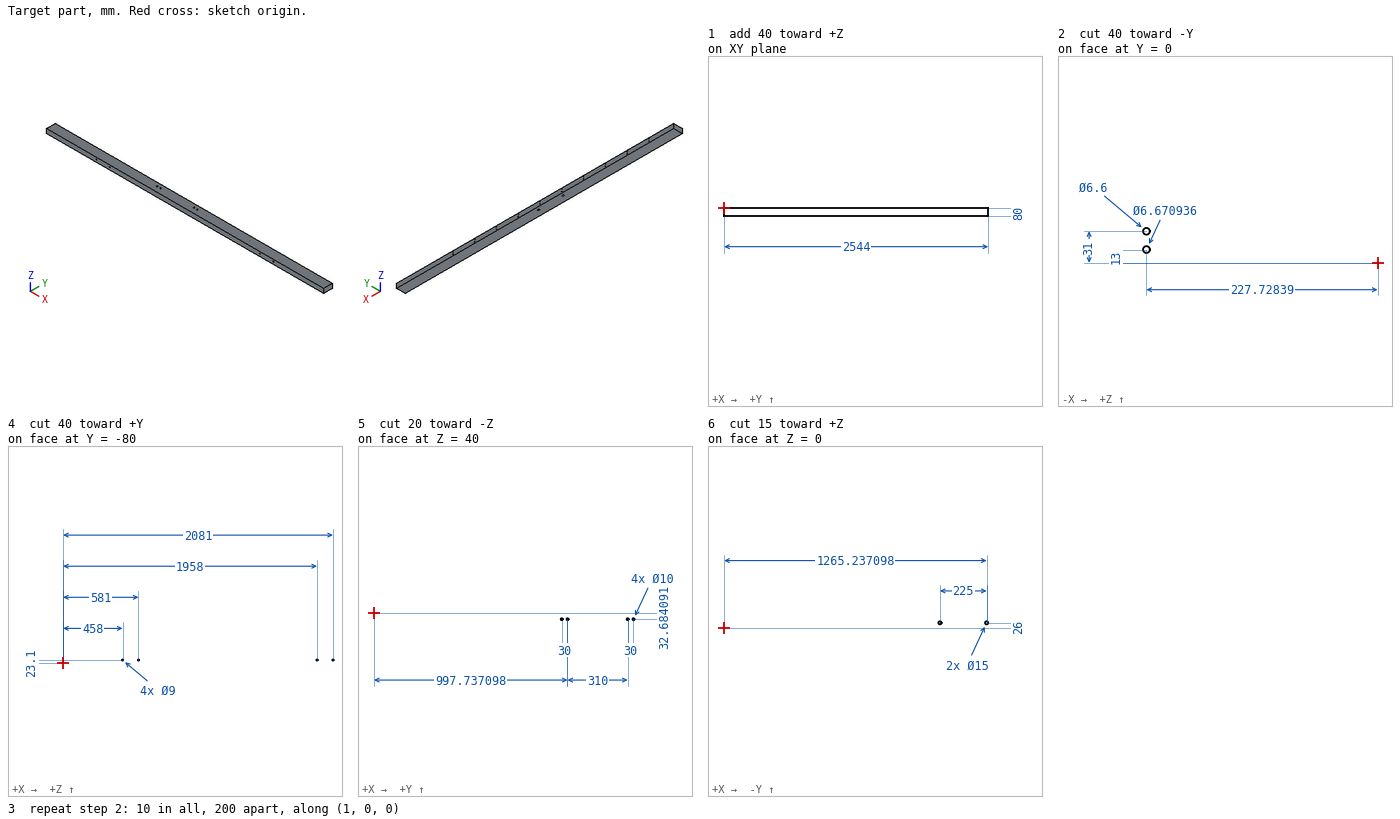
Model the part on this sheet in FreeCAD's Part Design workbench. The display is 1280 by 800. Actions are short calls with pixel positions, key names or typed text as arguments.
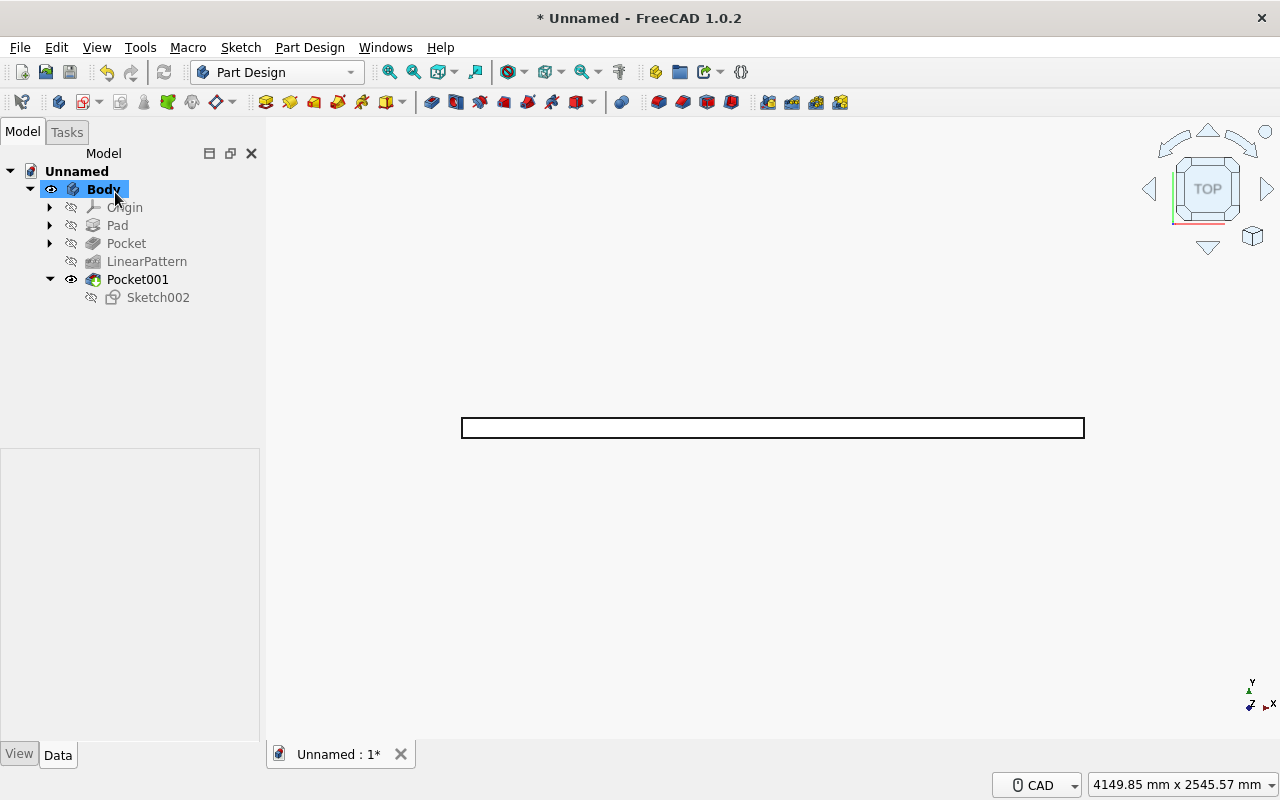
click(1039, 427)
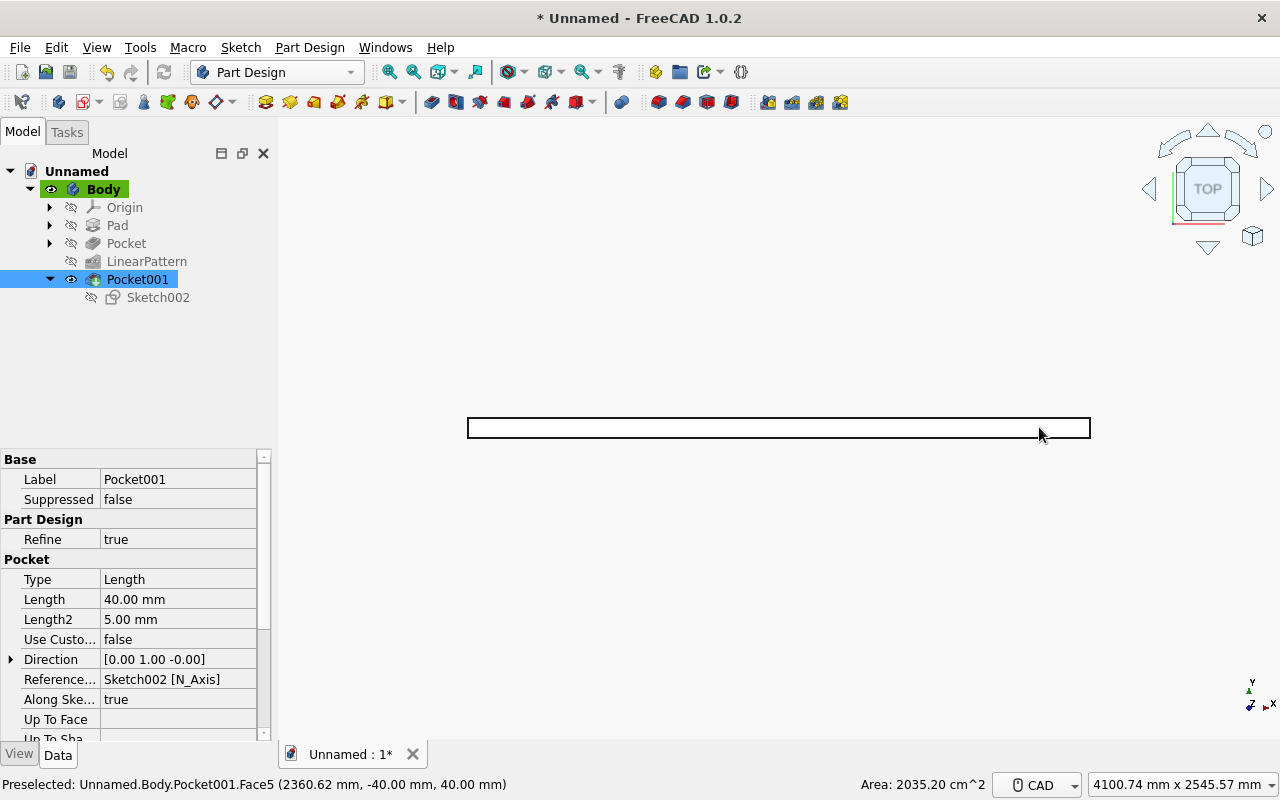
click(84, 102)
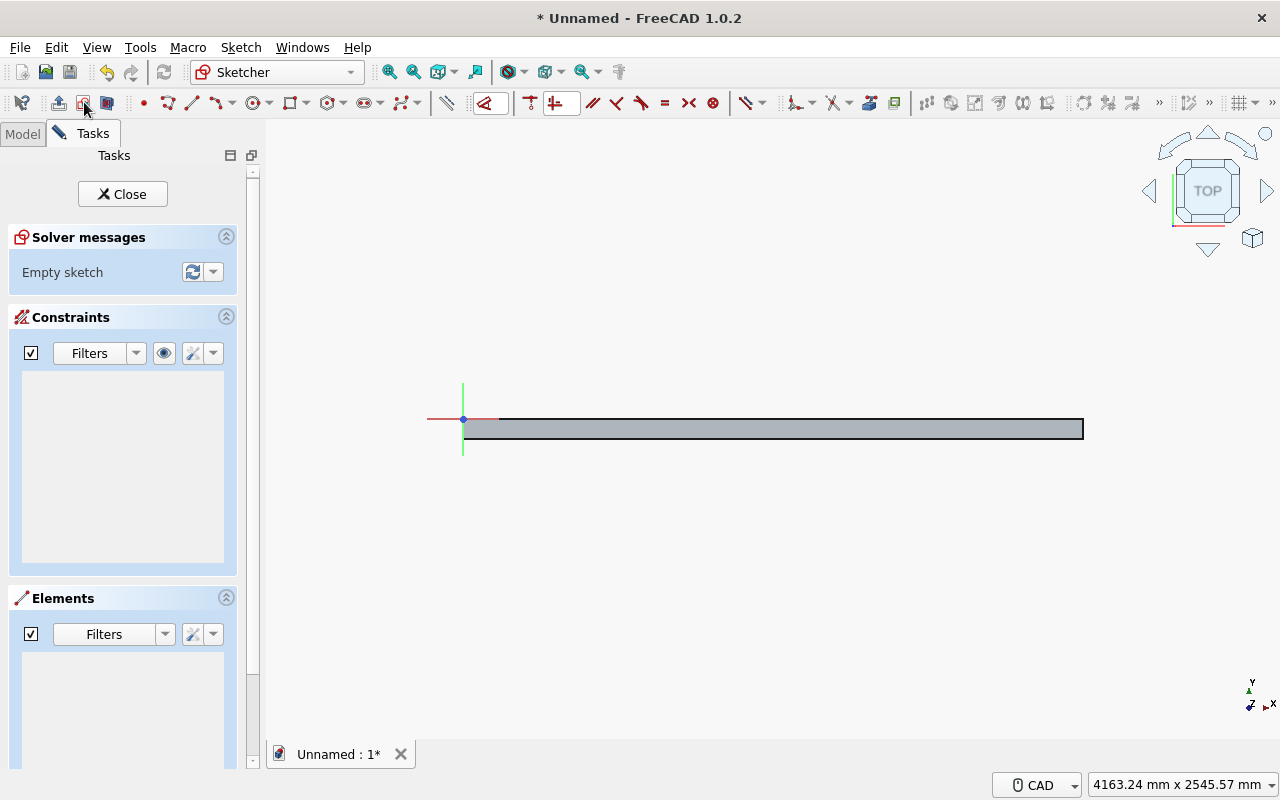
scroll(752, 427, up, 9)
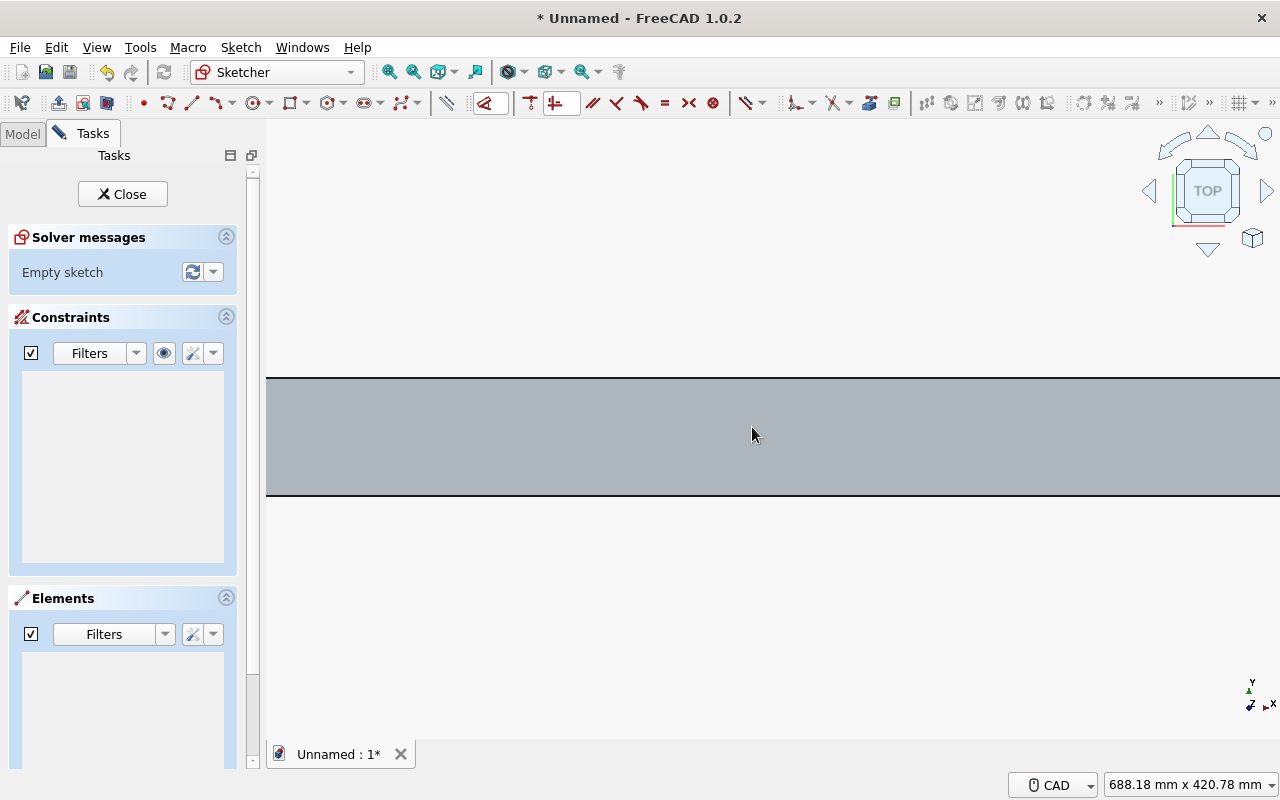
click(254, 104)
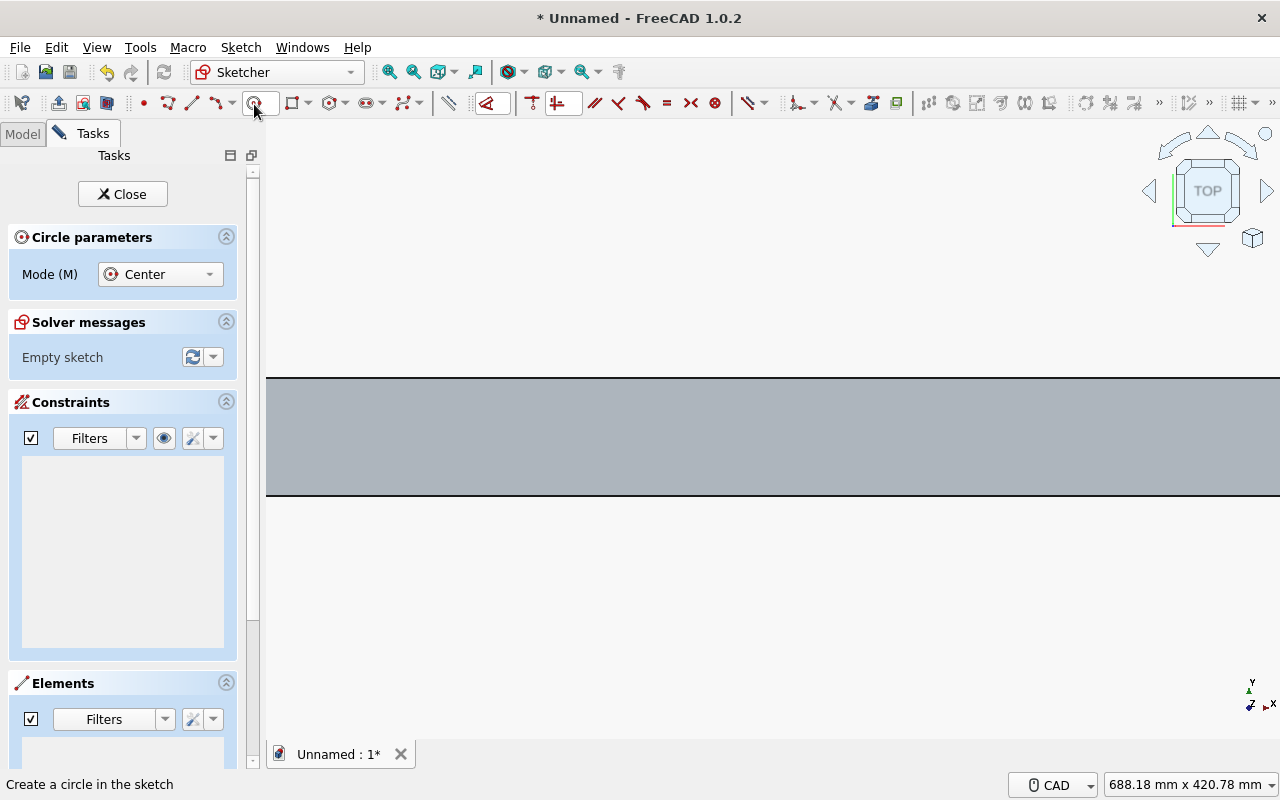
scroll(973, 426, up, 6)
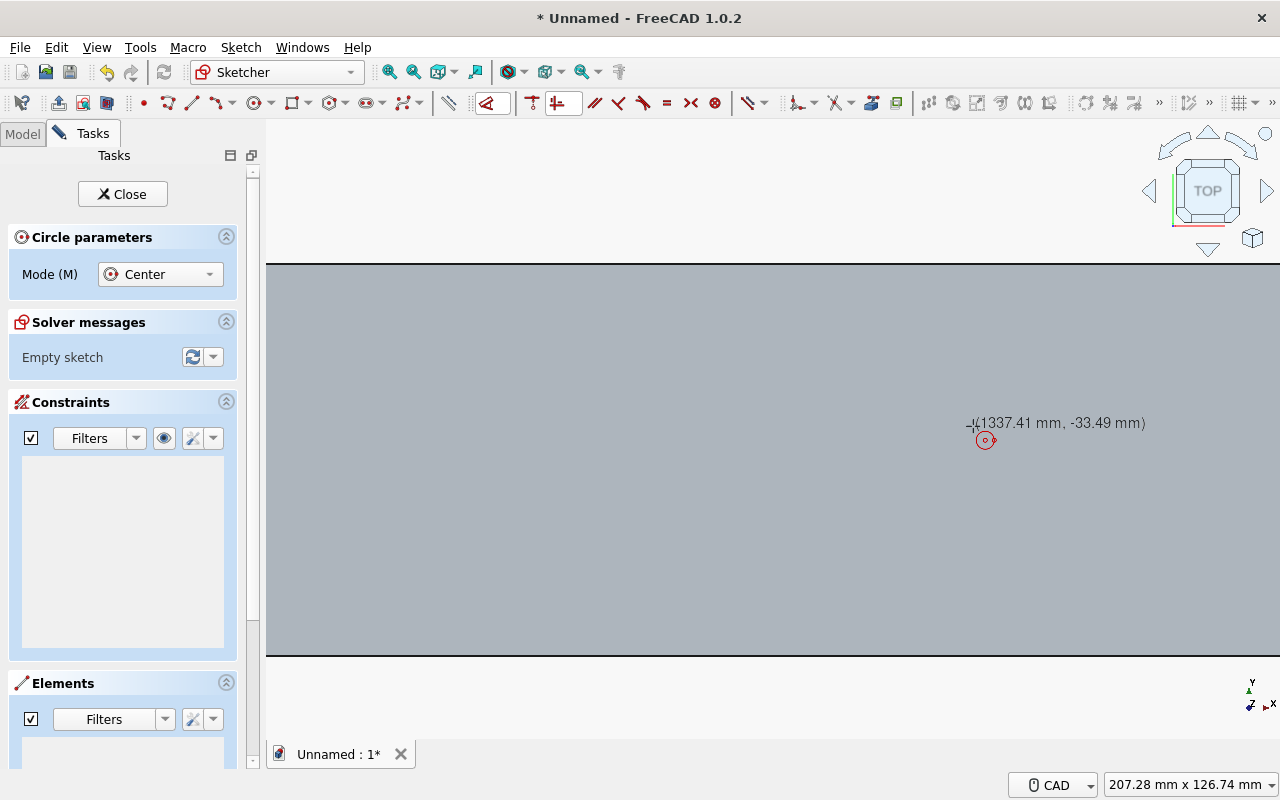
click(973, 424)
move(990, 407)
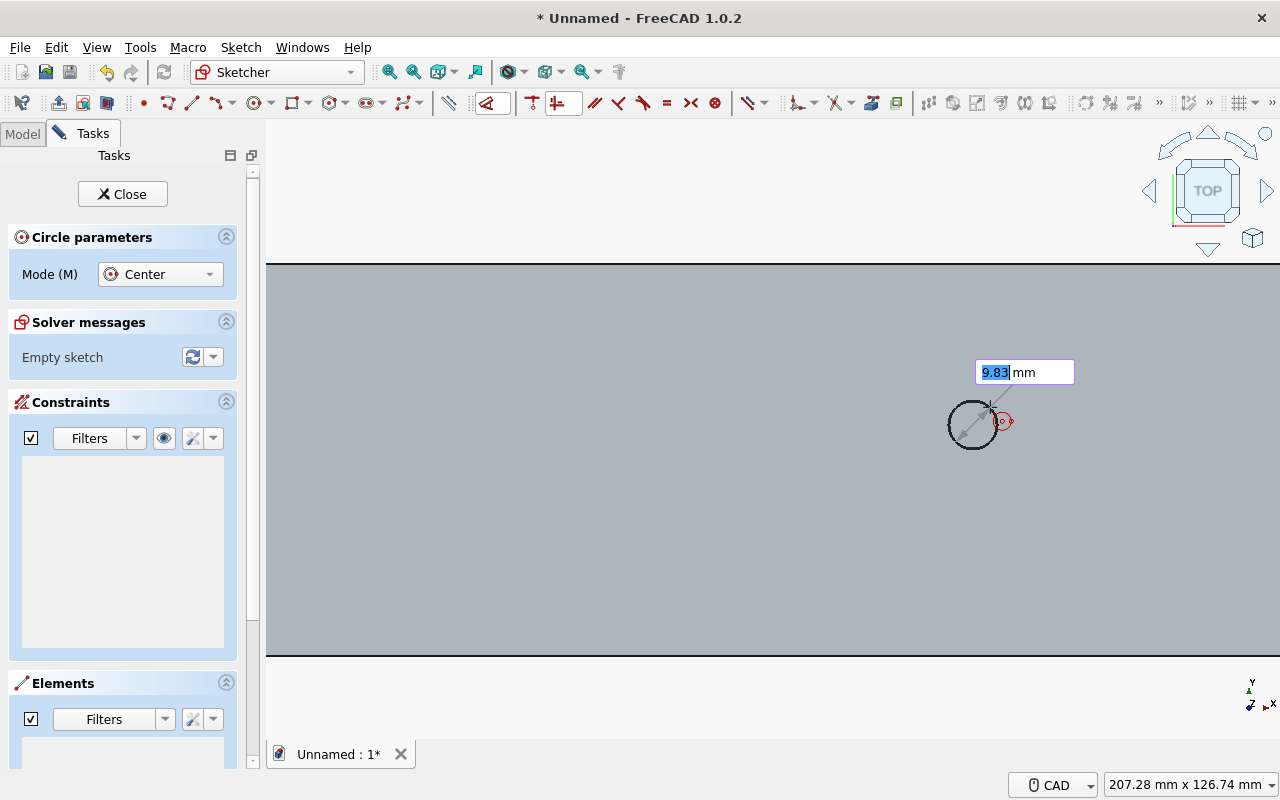
text(10)
key(Return)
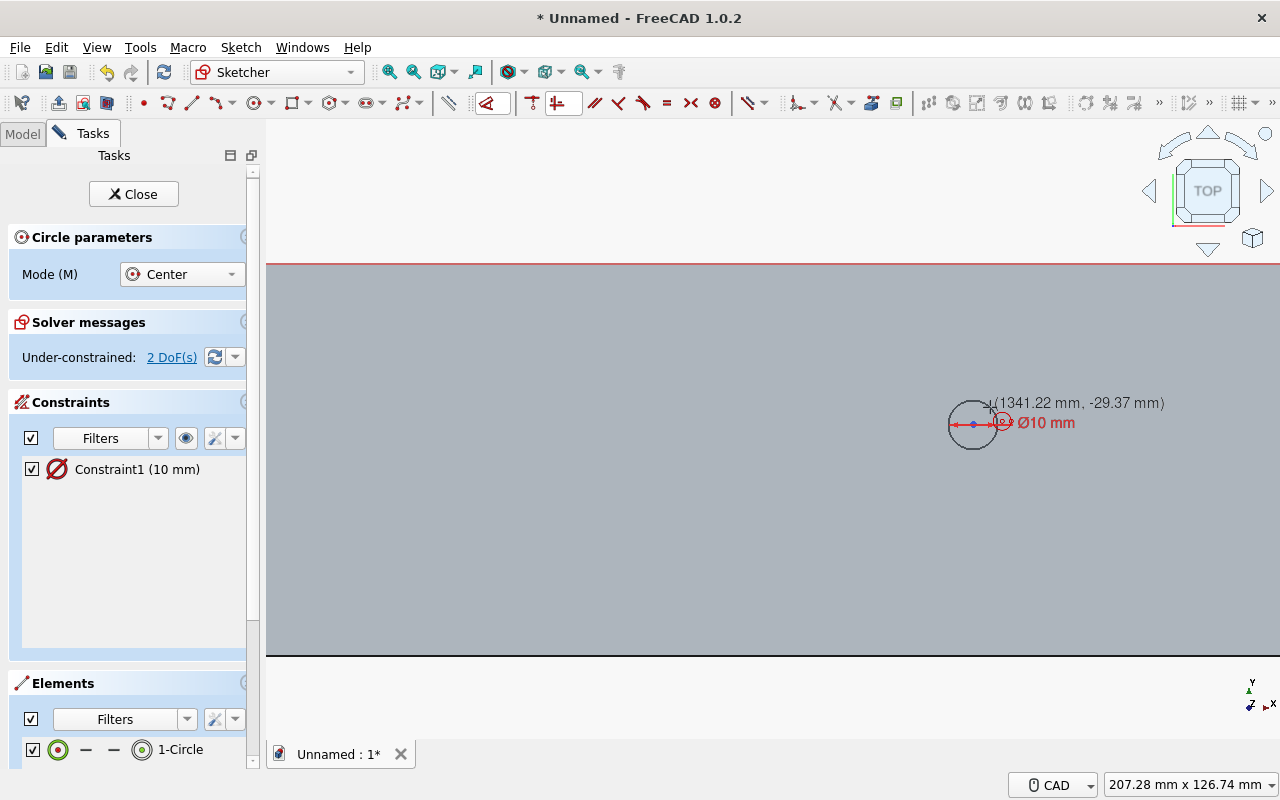
click(826, 424)
move(844, 407)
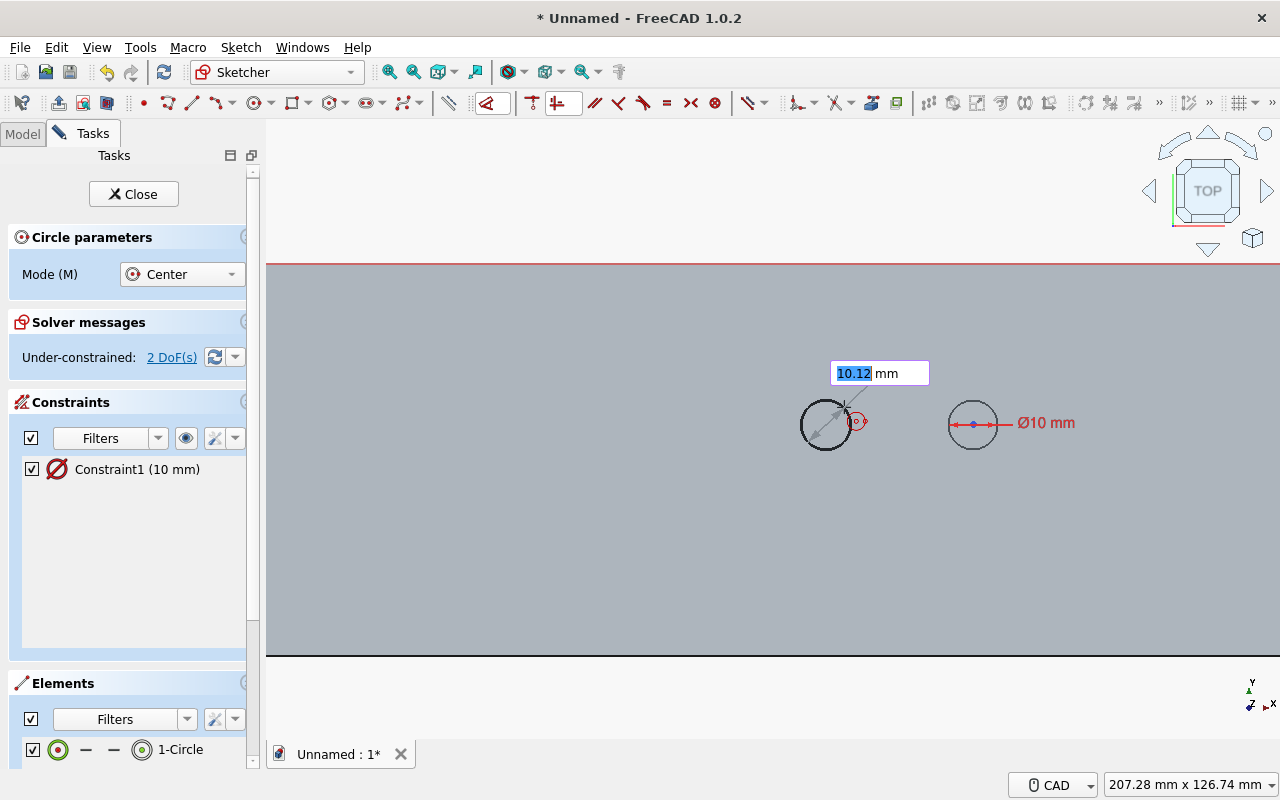
text(10)
key(Return)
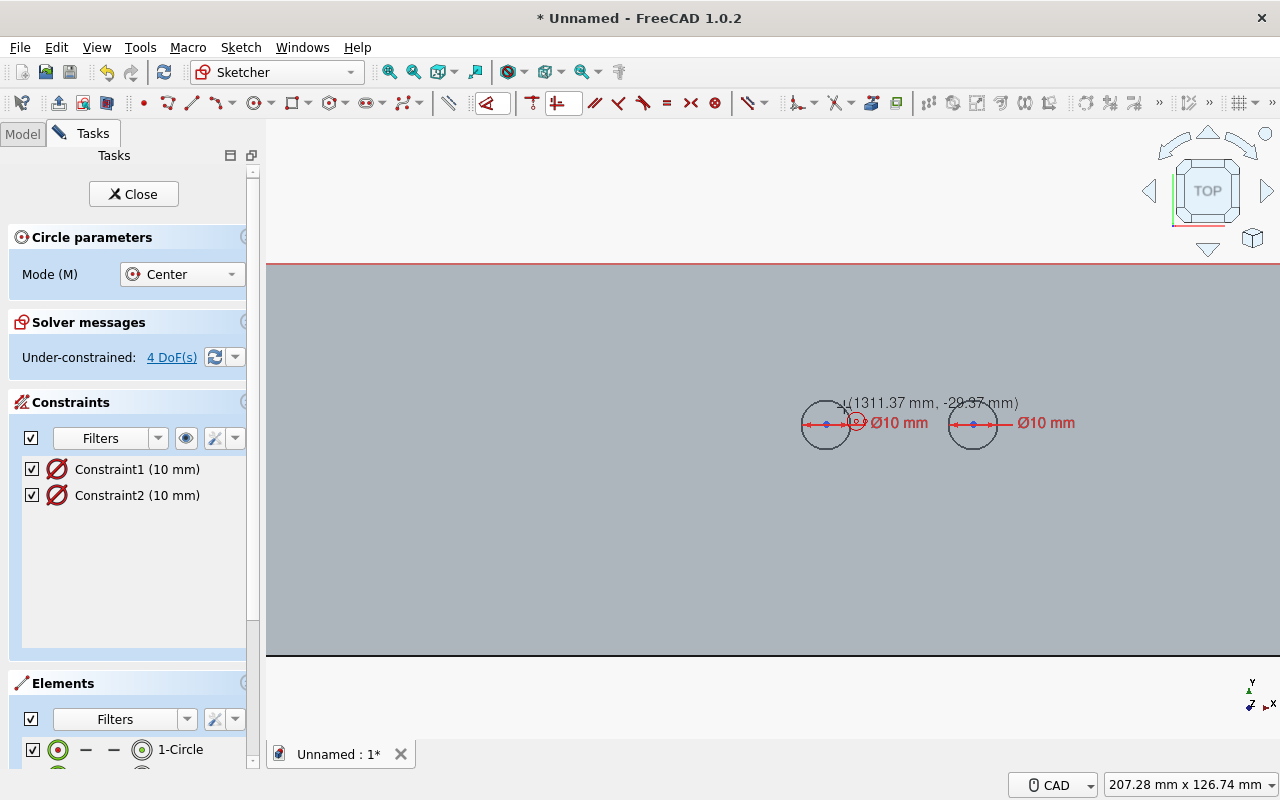
scroll(979, 431, down, 6)